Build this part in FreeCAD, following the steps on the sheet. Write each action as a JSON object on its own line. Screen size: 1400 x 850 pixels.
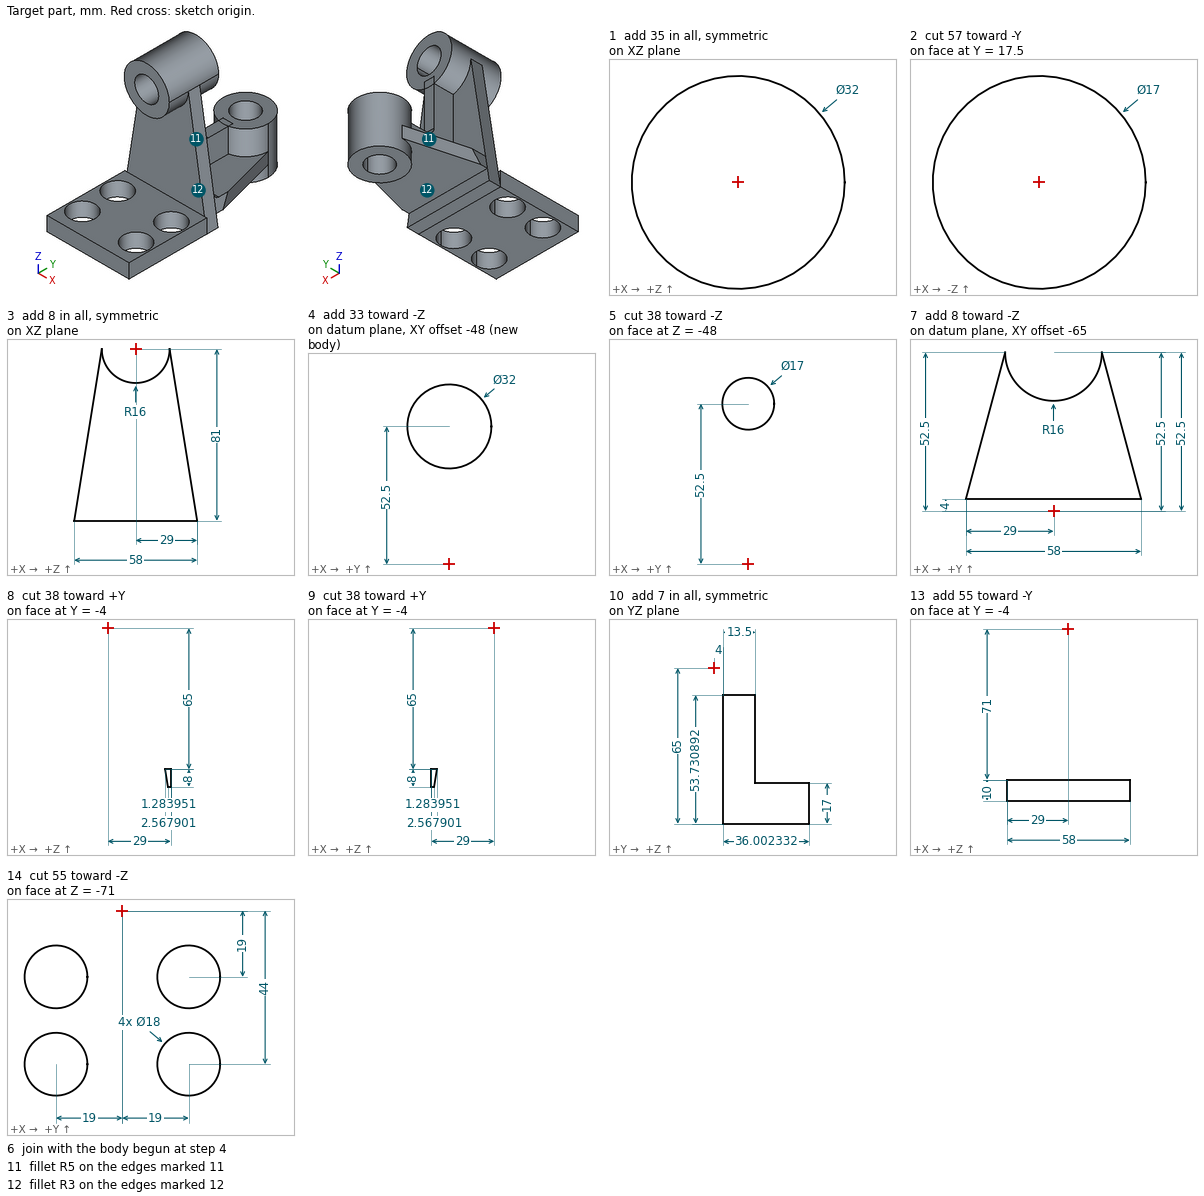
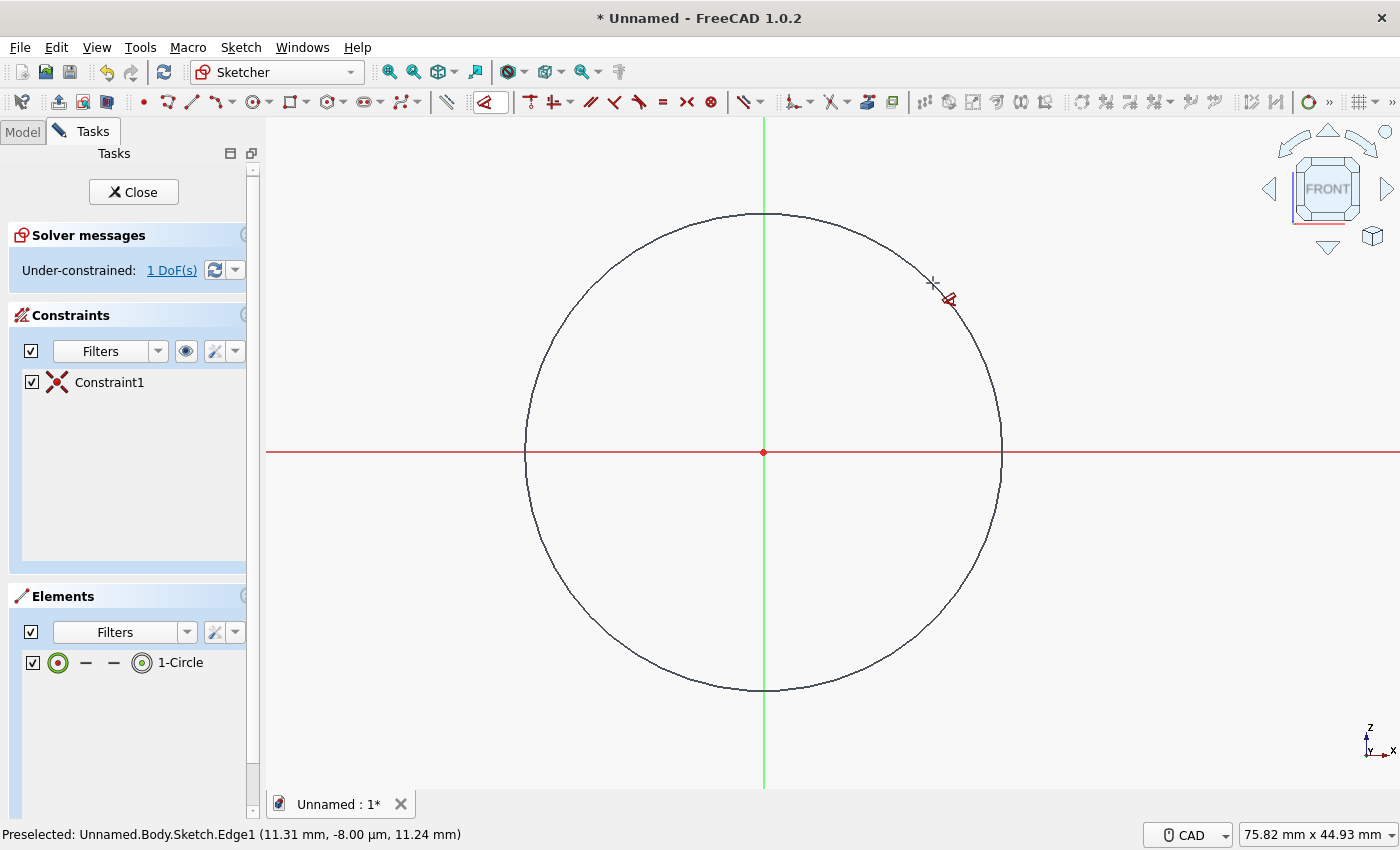
{"action": "left_click", "coordinate": [932, 283]}
{"action": "left_click", "coordinate": [955, 260]}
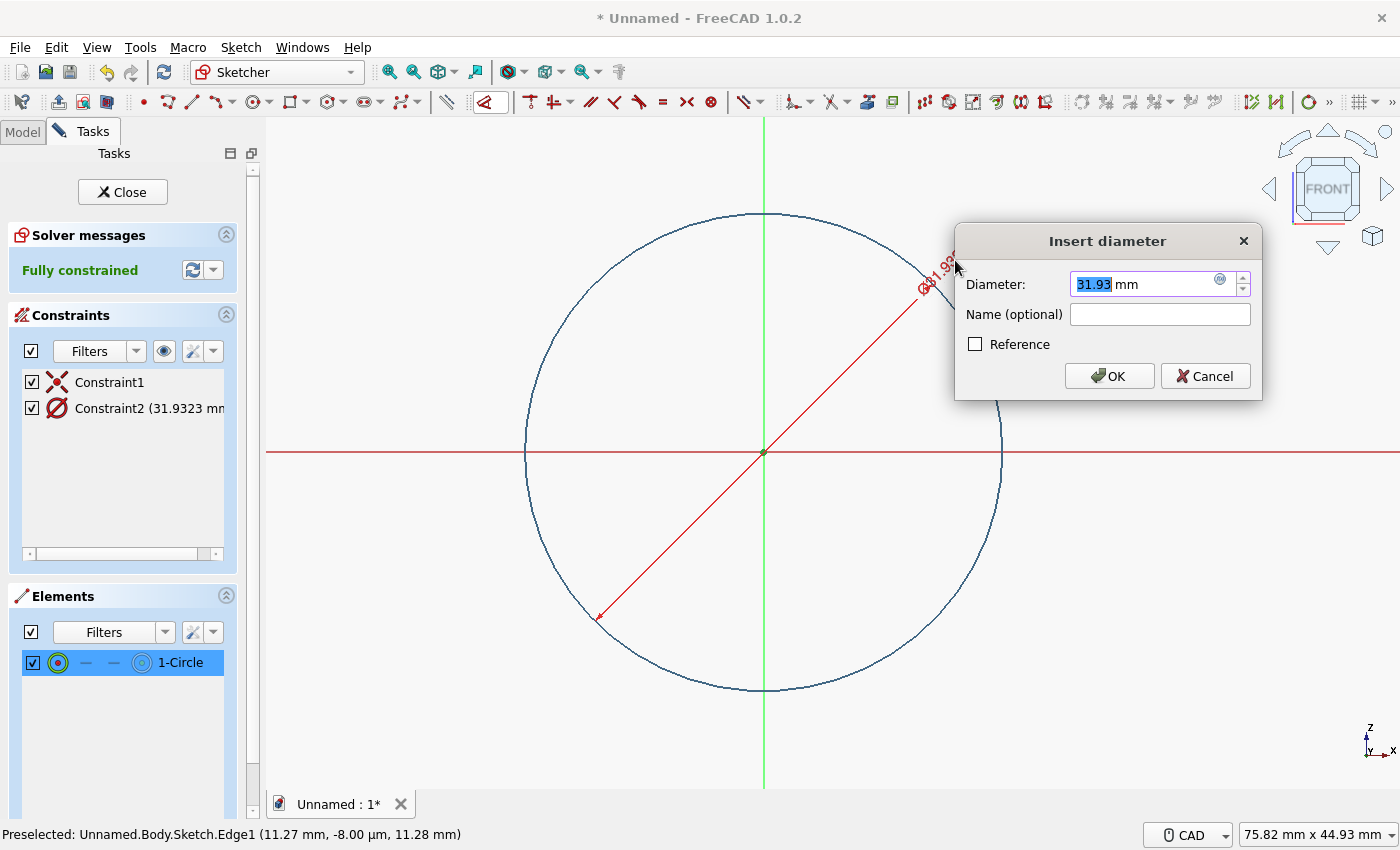
{"action": "type", "text": "32"}
{"action": "key", "text": "Return"}
{"action": "key", "text": "Escape"}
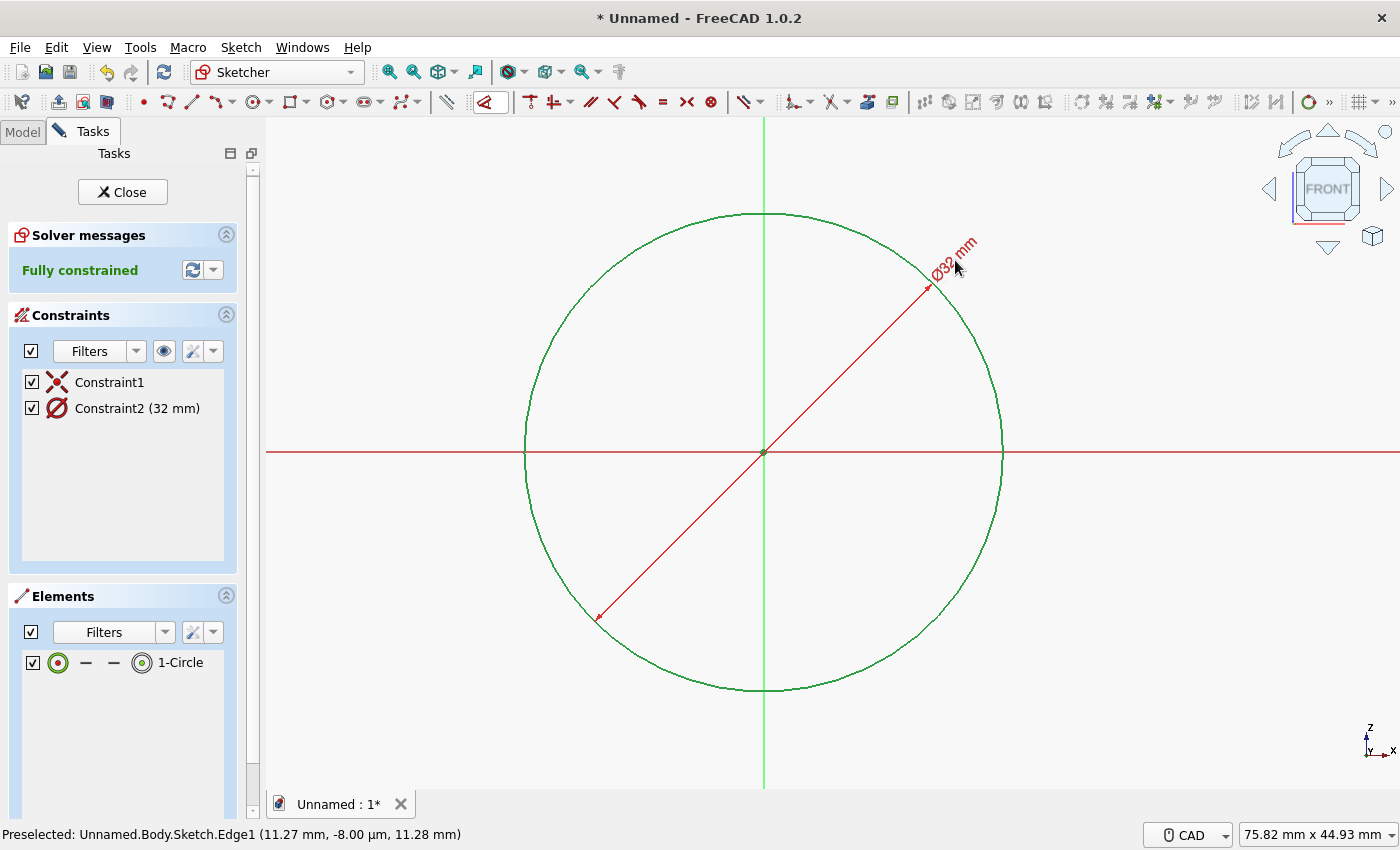
{"action": "left_click", "coordinate": [123, 192]}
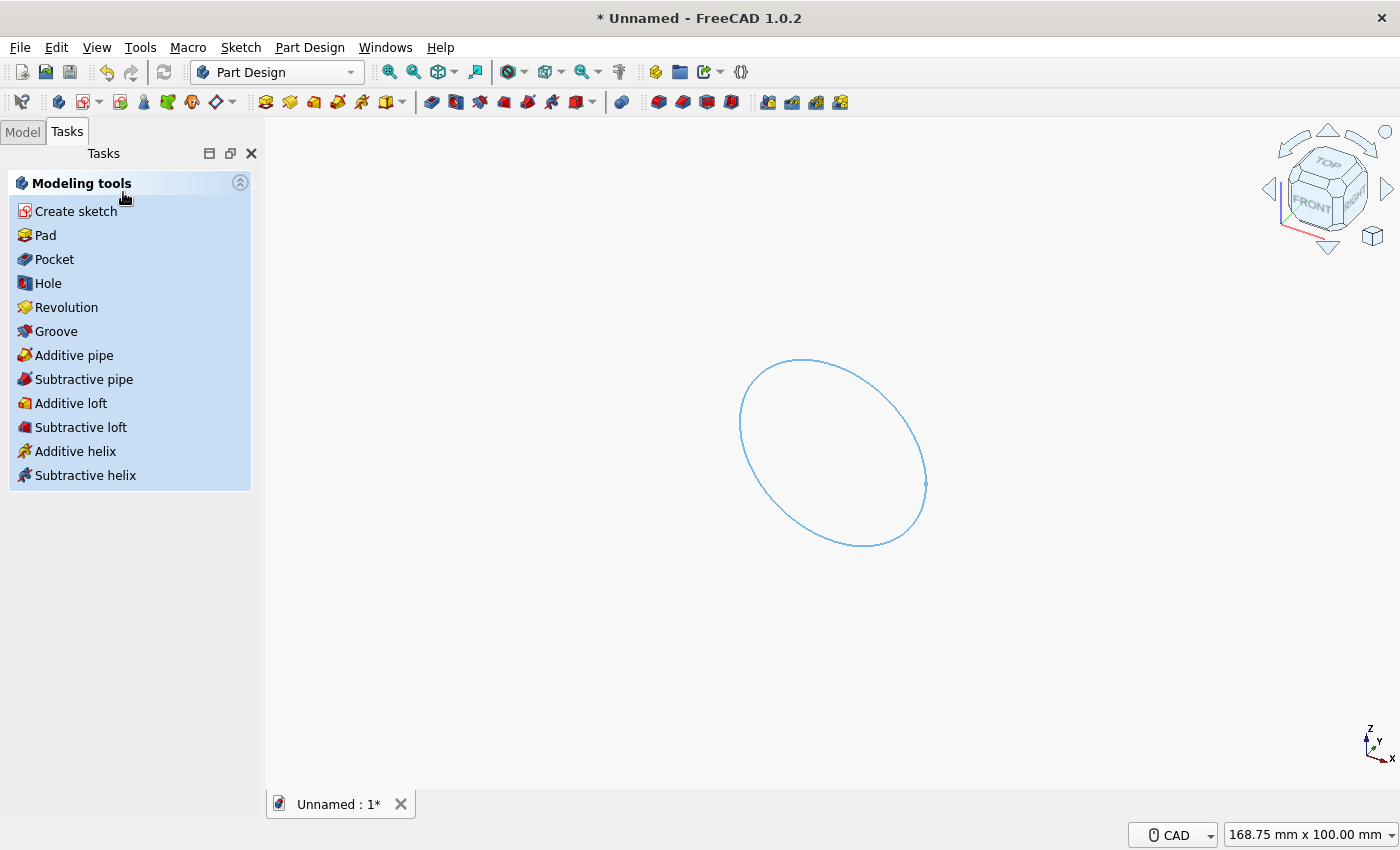
{"action": "left_click", "coordinate": [266, 102]}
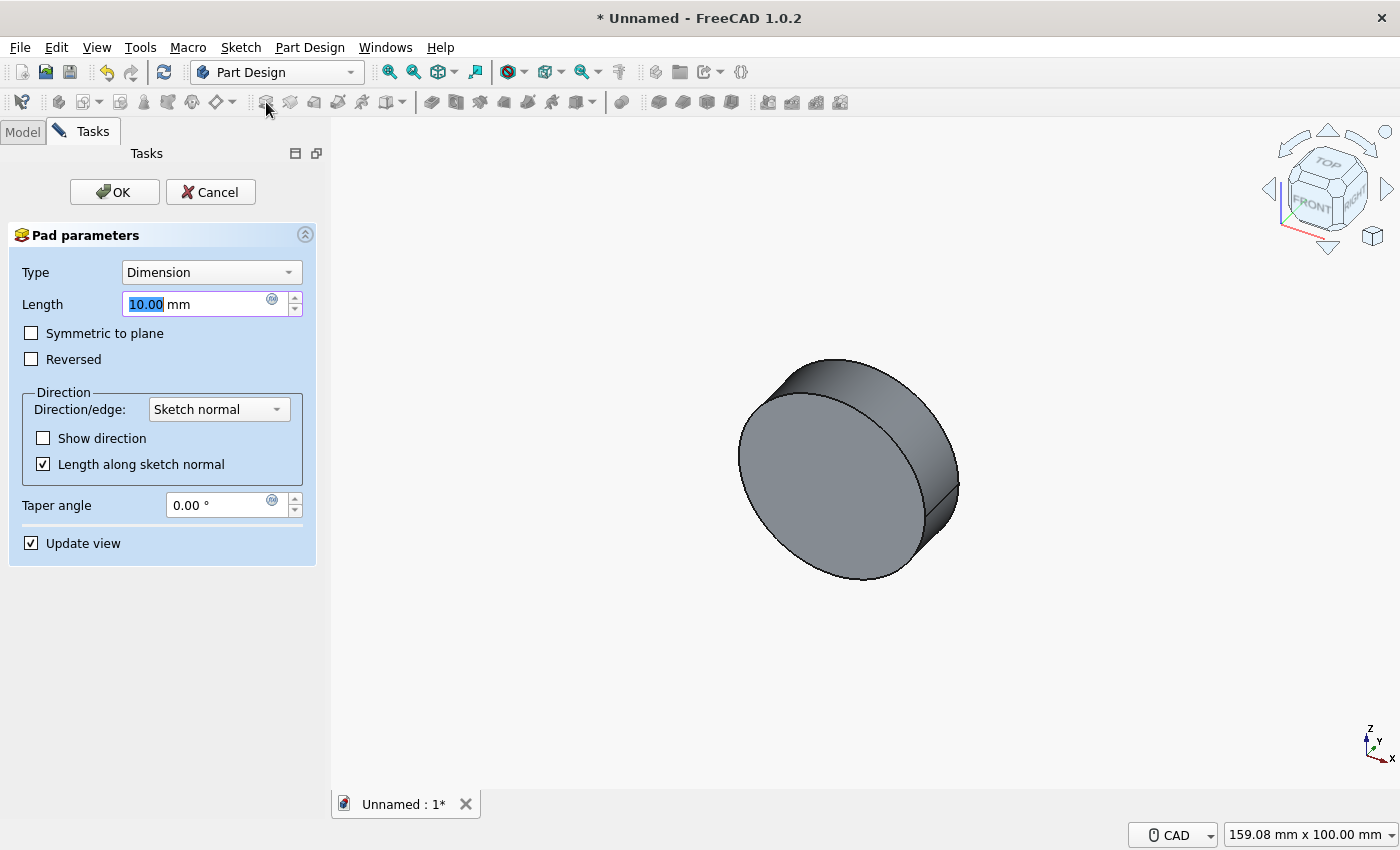
{"action": "type", "text": "35"}
{"action": "key", "text": "Tab"}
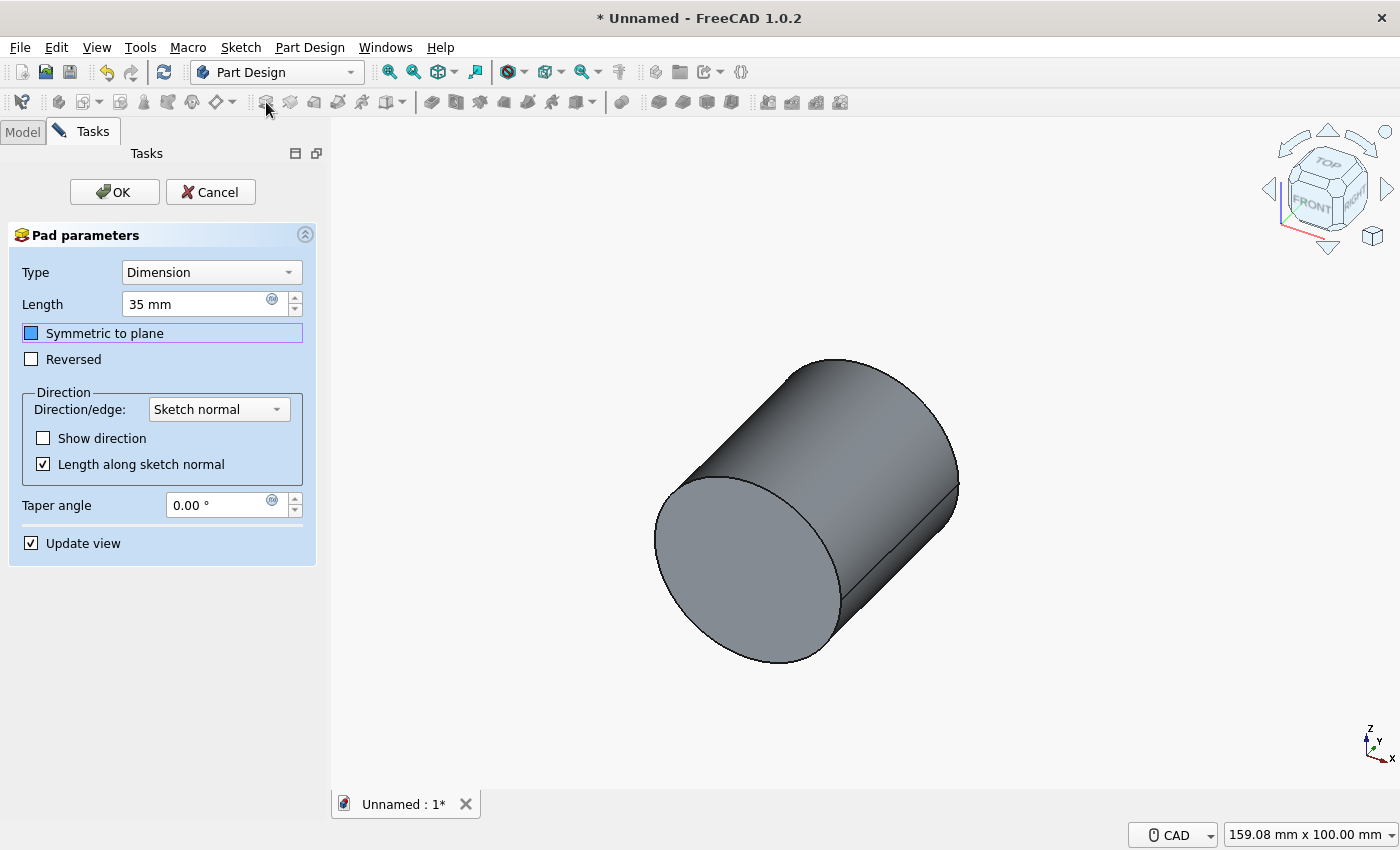
{"action": "left_click", "coordinate": [30, 333]}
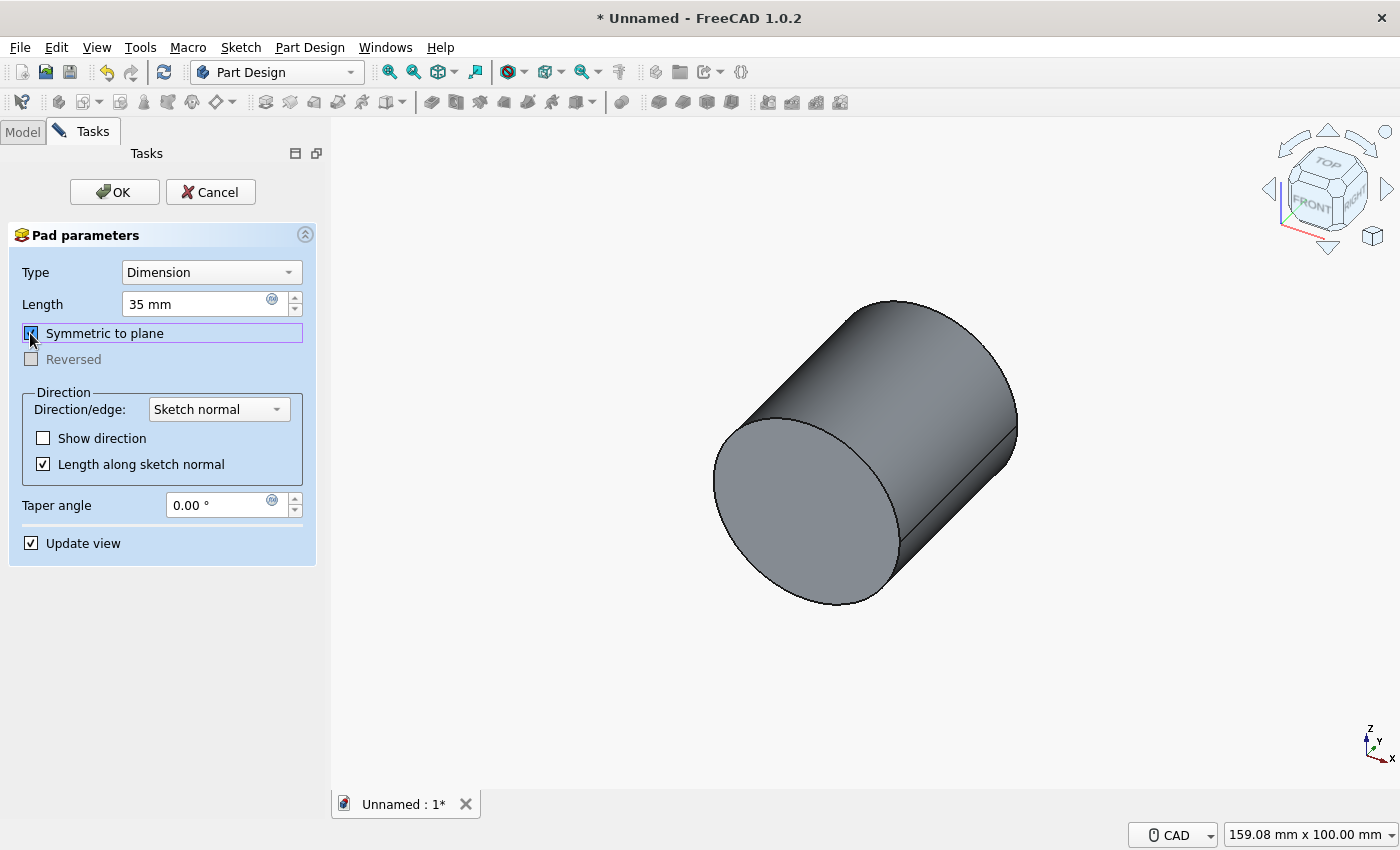
{"action": "left_click", "coordinate": [115, 192]}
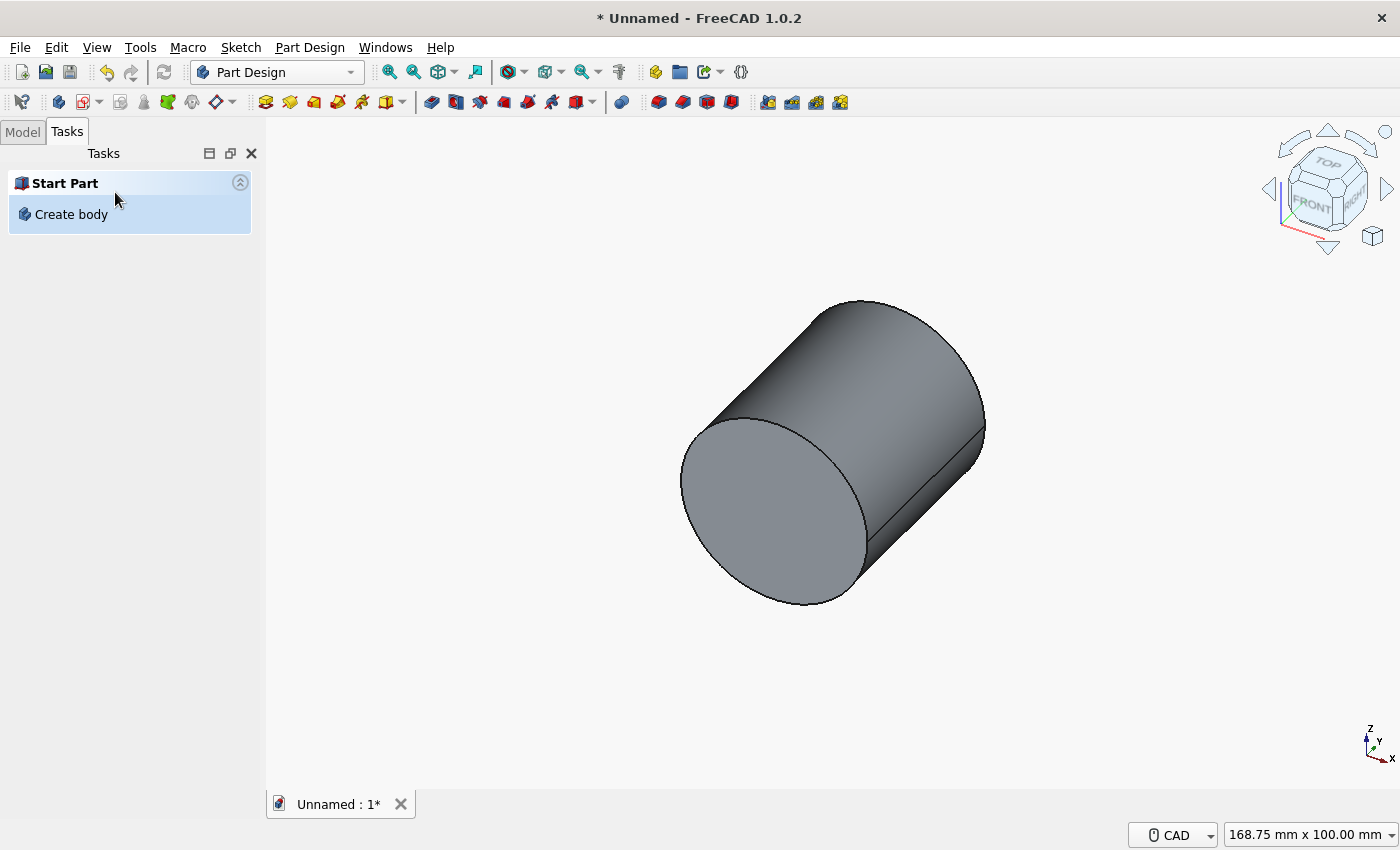
{"action": "key", "text": "4"}